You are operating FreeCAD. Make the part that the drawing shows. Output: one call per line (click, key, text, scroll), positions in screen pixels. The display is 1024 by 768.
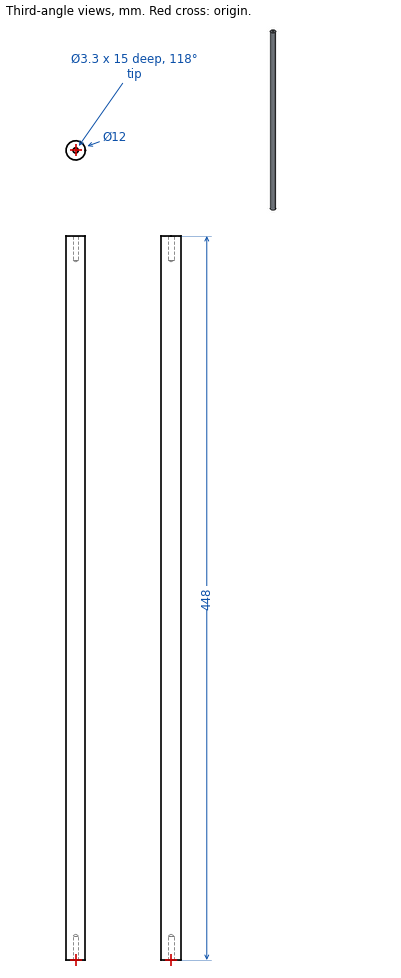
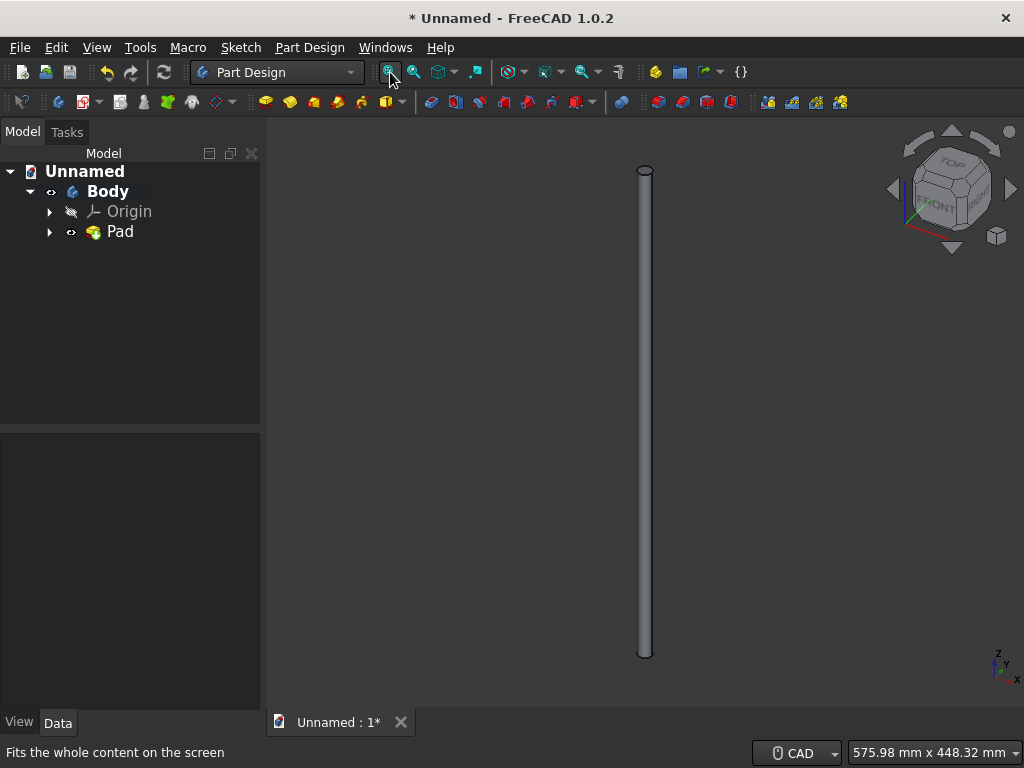
key(5)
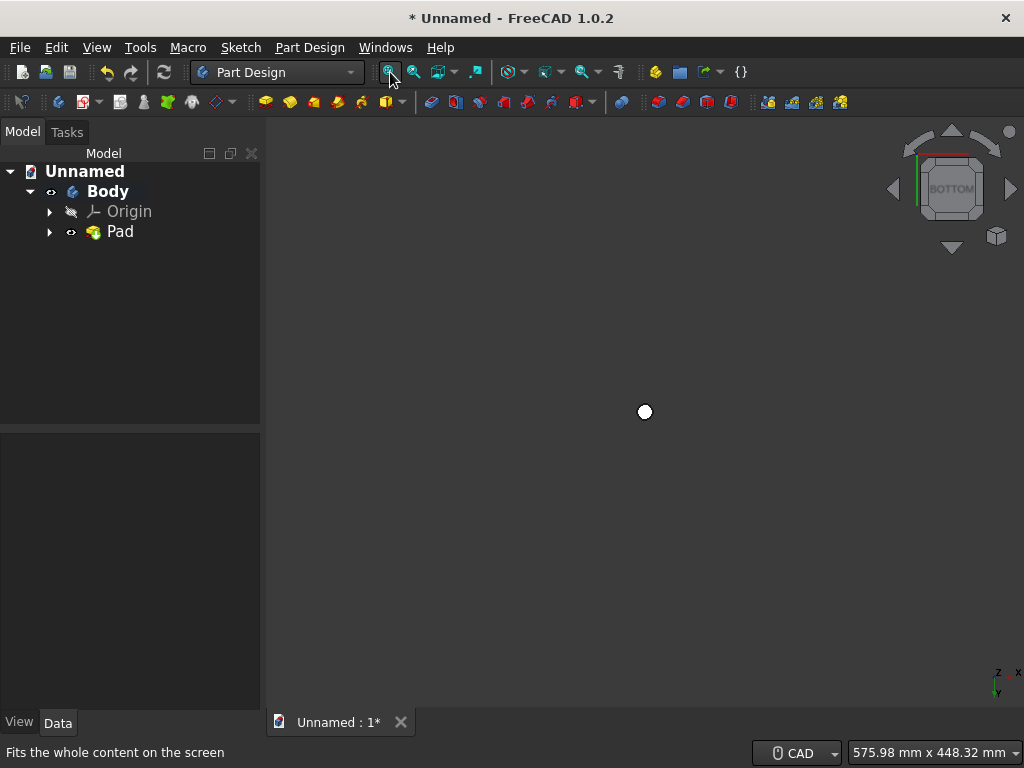
click(390, 72)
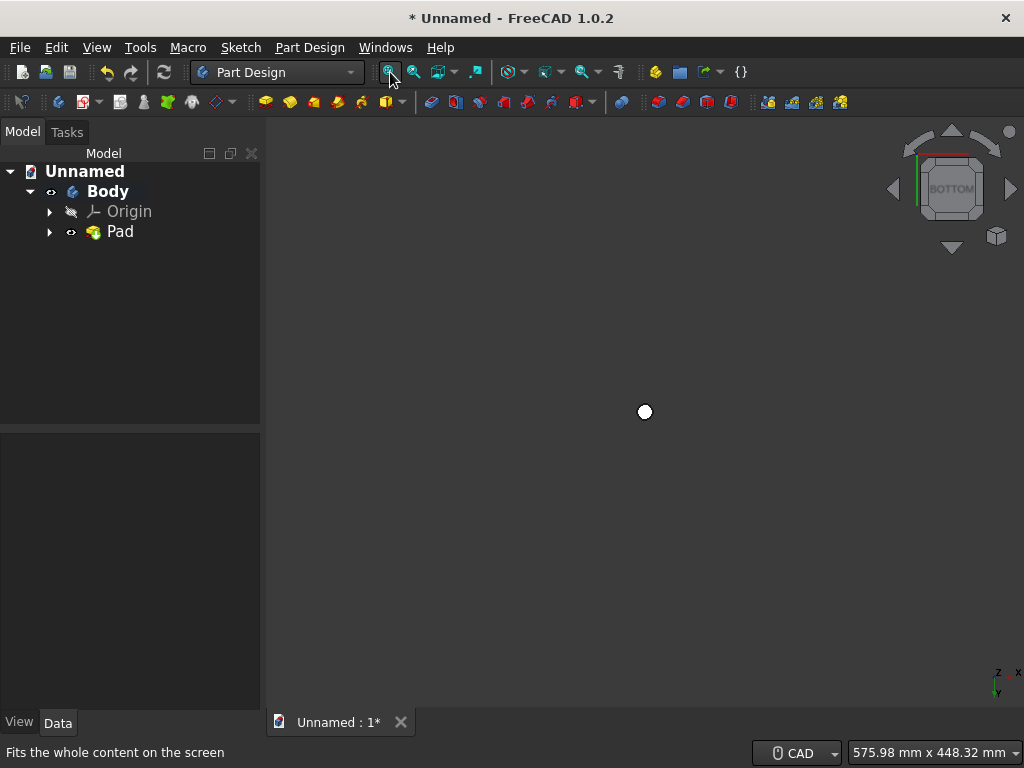
key(1)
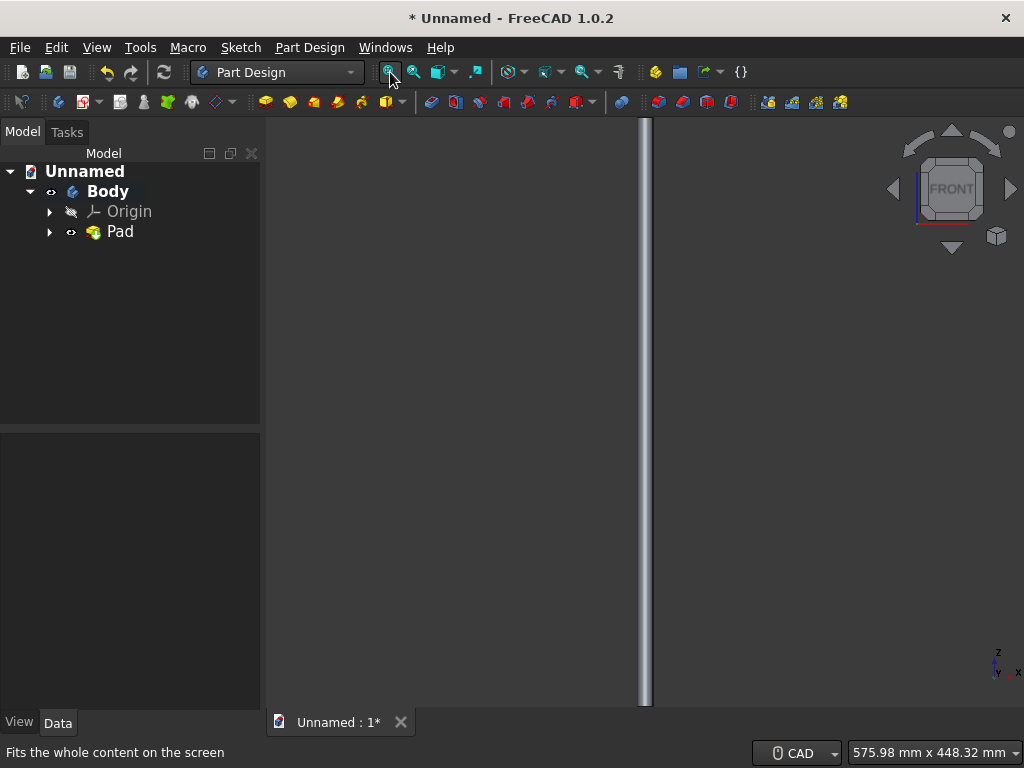
click(390, 72)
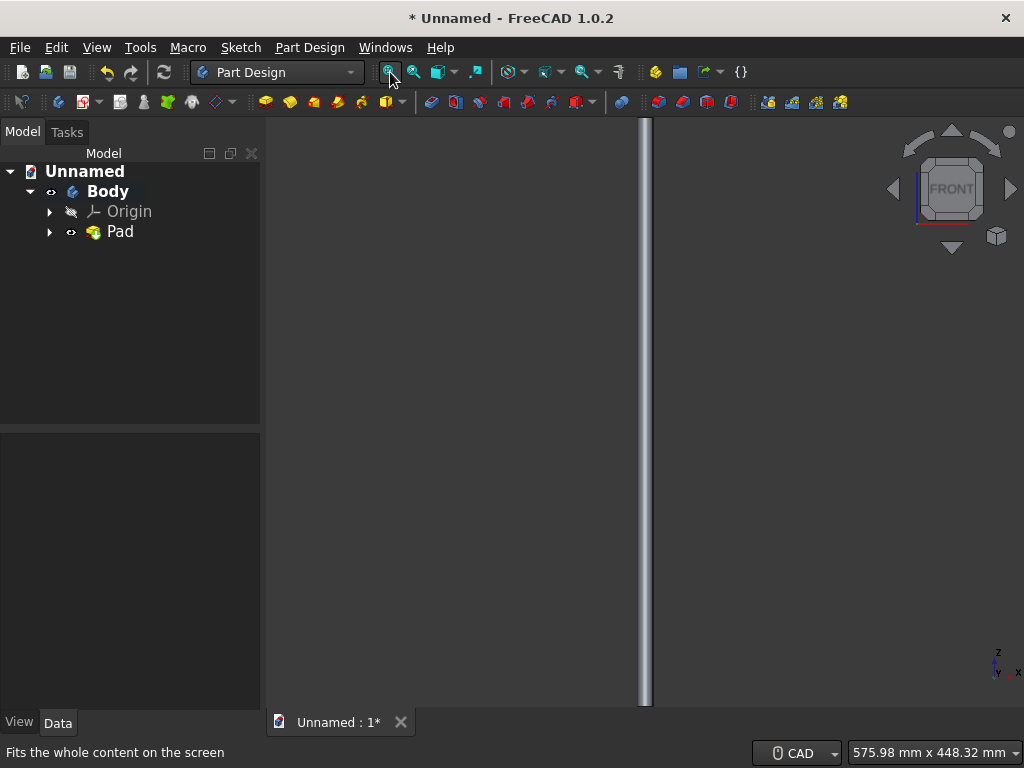
key(3)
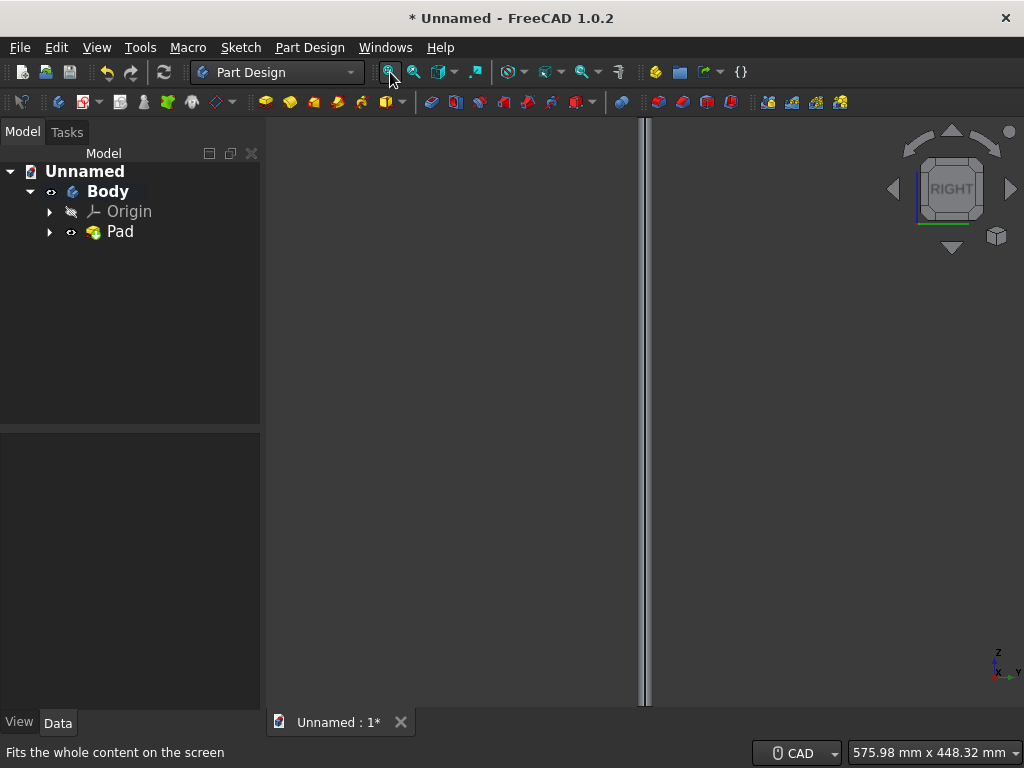
click(390, 72)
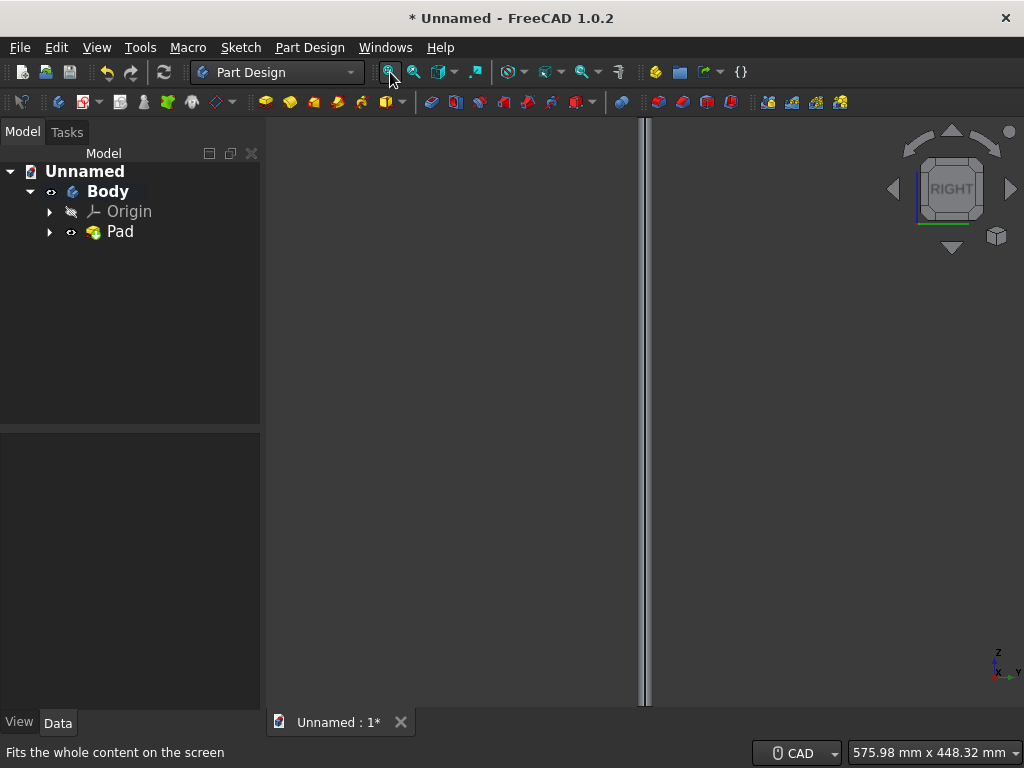
click(84, 102)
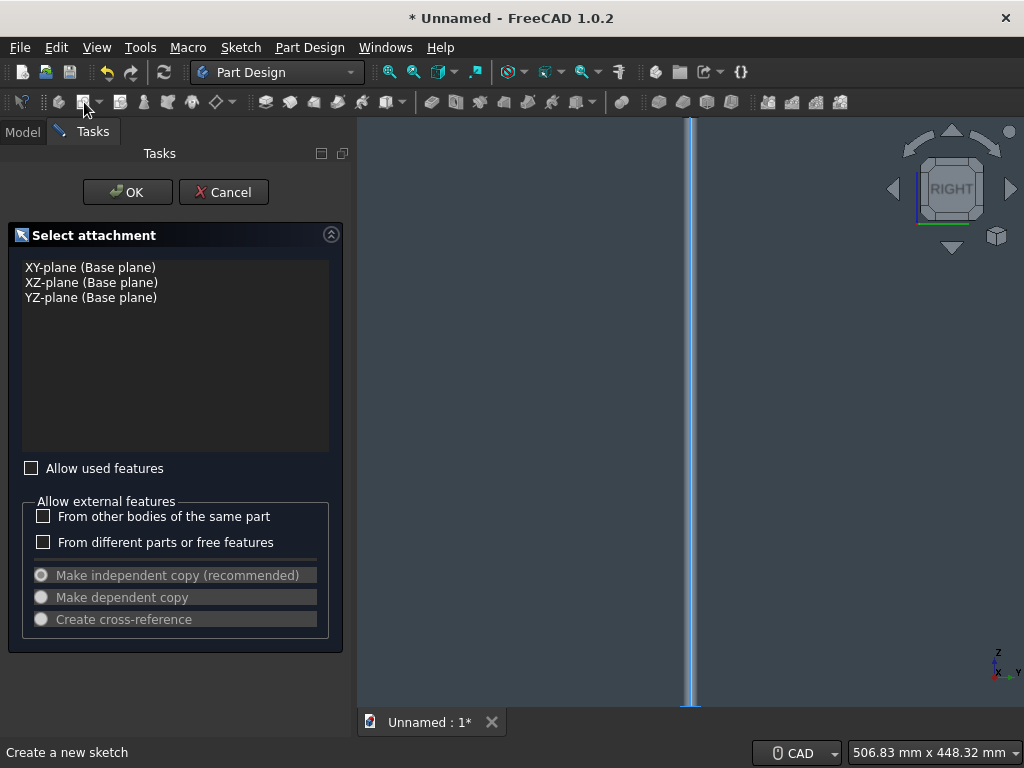
click(82, 268)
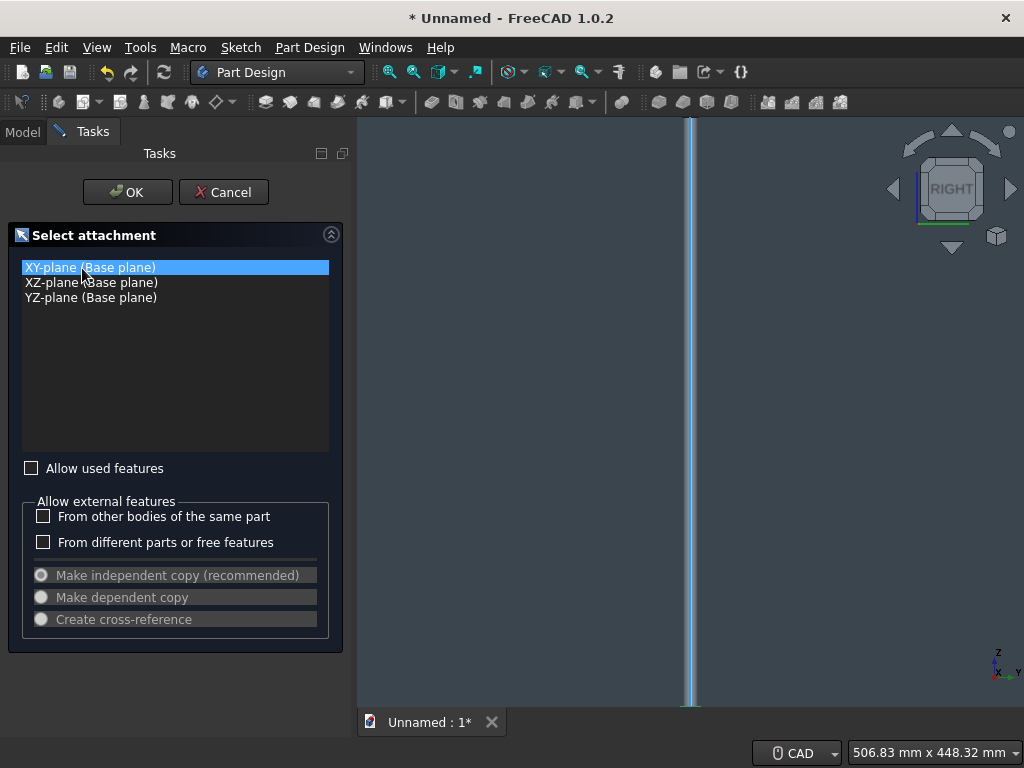
click(128, 192)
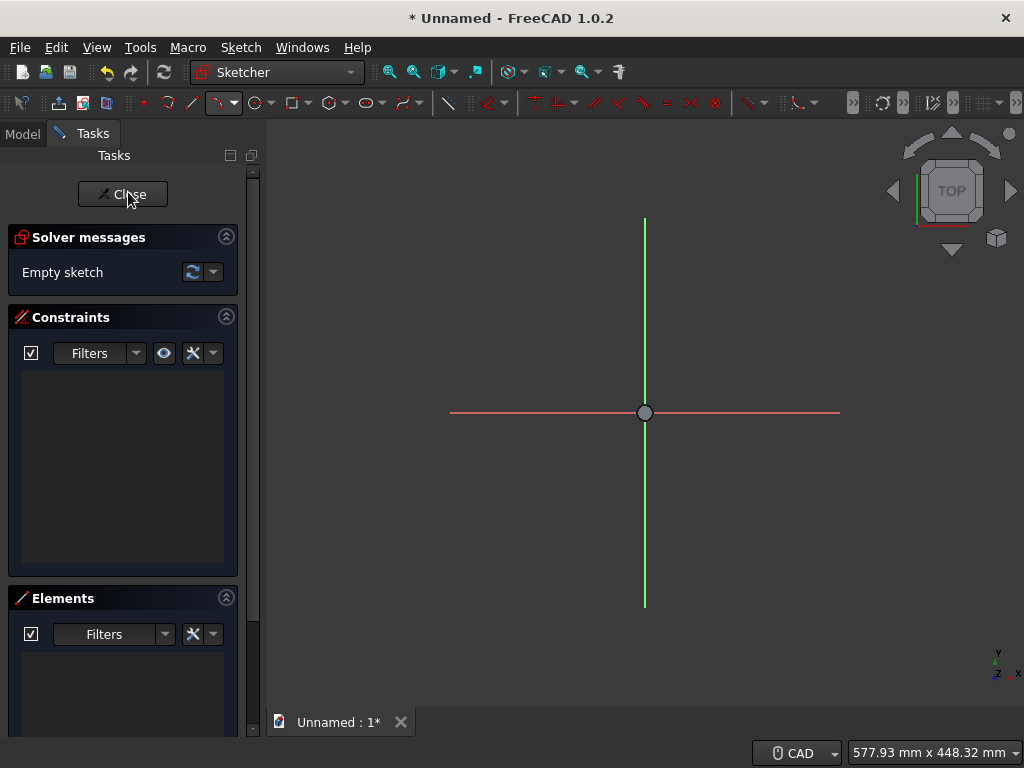
click(108, 104)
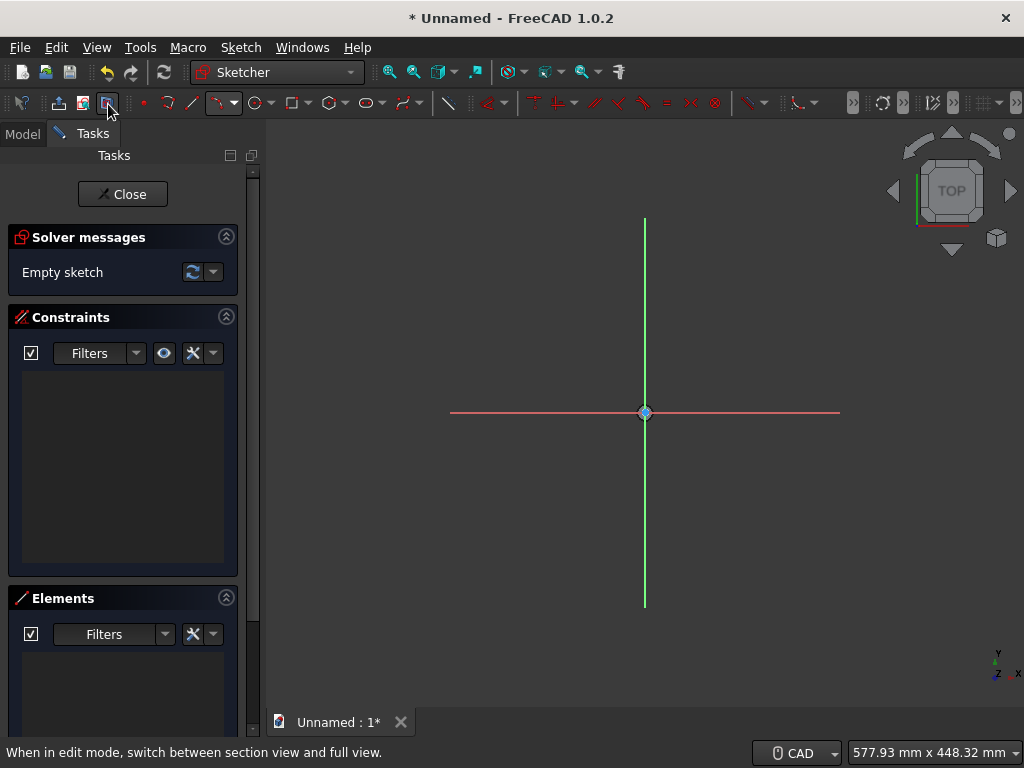
scroll(649, 413, up, 15)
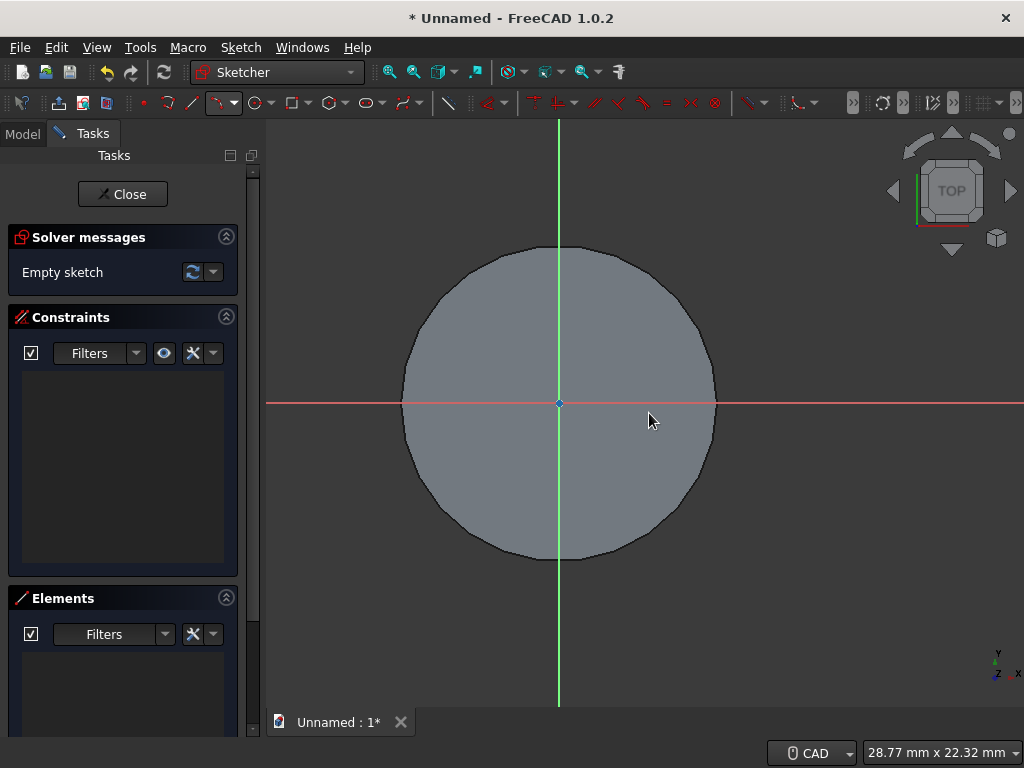
scroll(553, 400, up, 7)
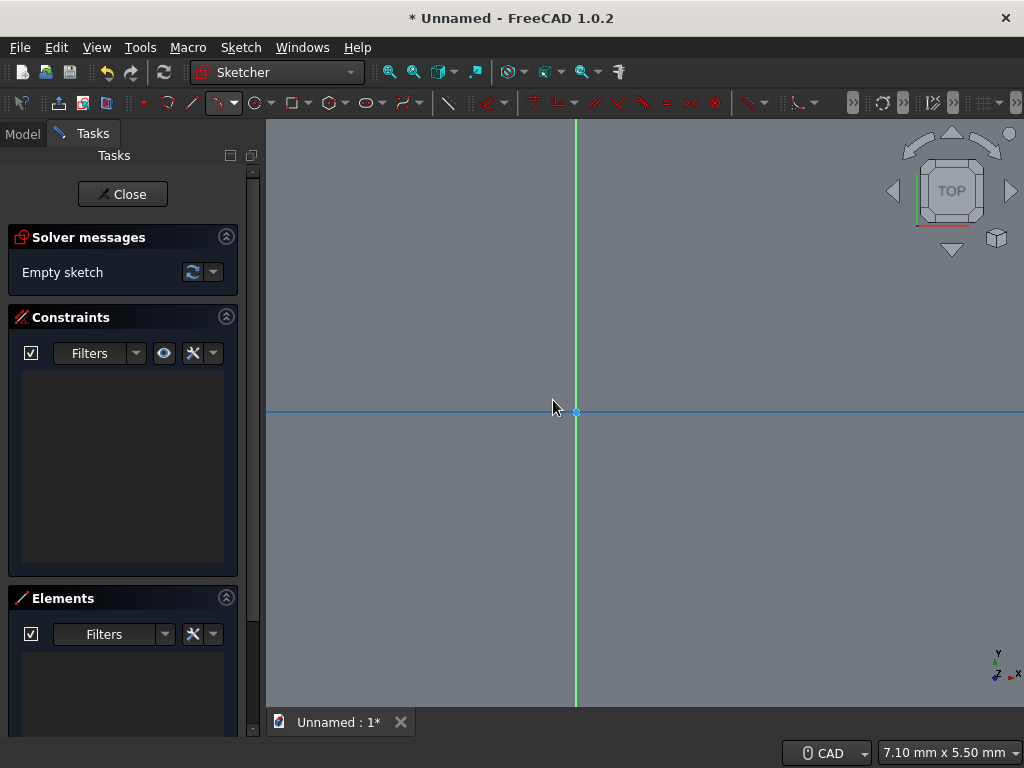
click(256, 104)